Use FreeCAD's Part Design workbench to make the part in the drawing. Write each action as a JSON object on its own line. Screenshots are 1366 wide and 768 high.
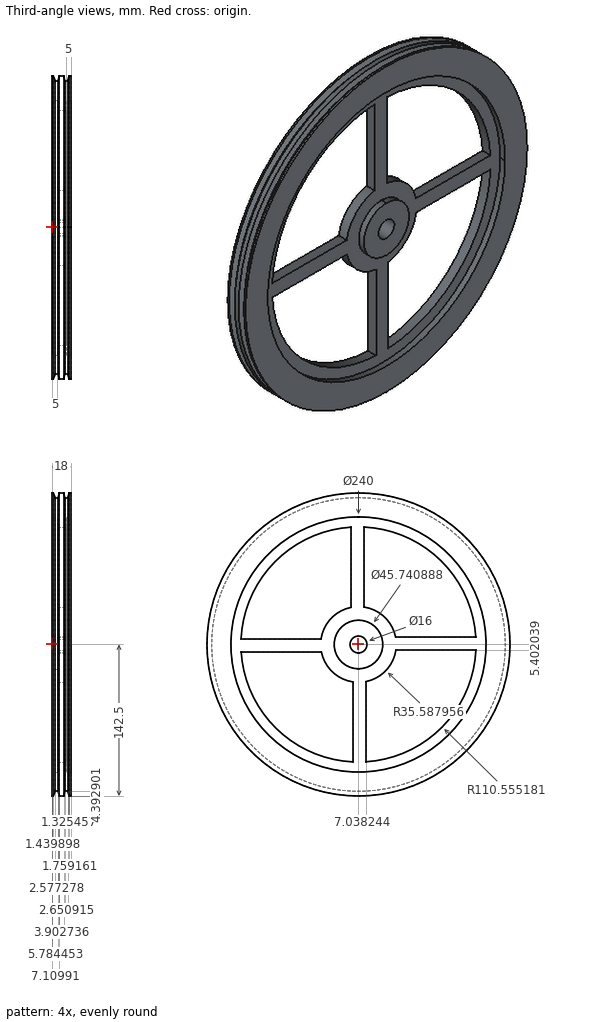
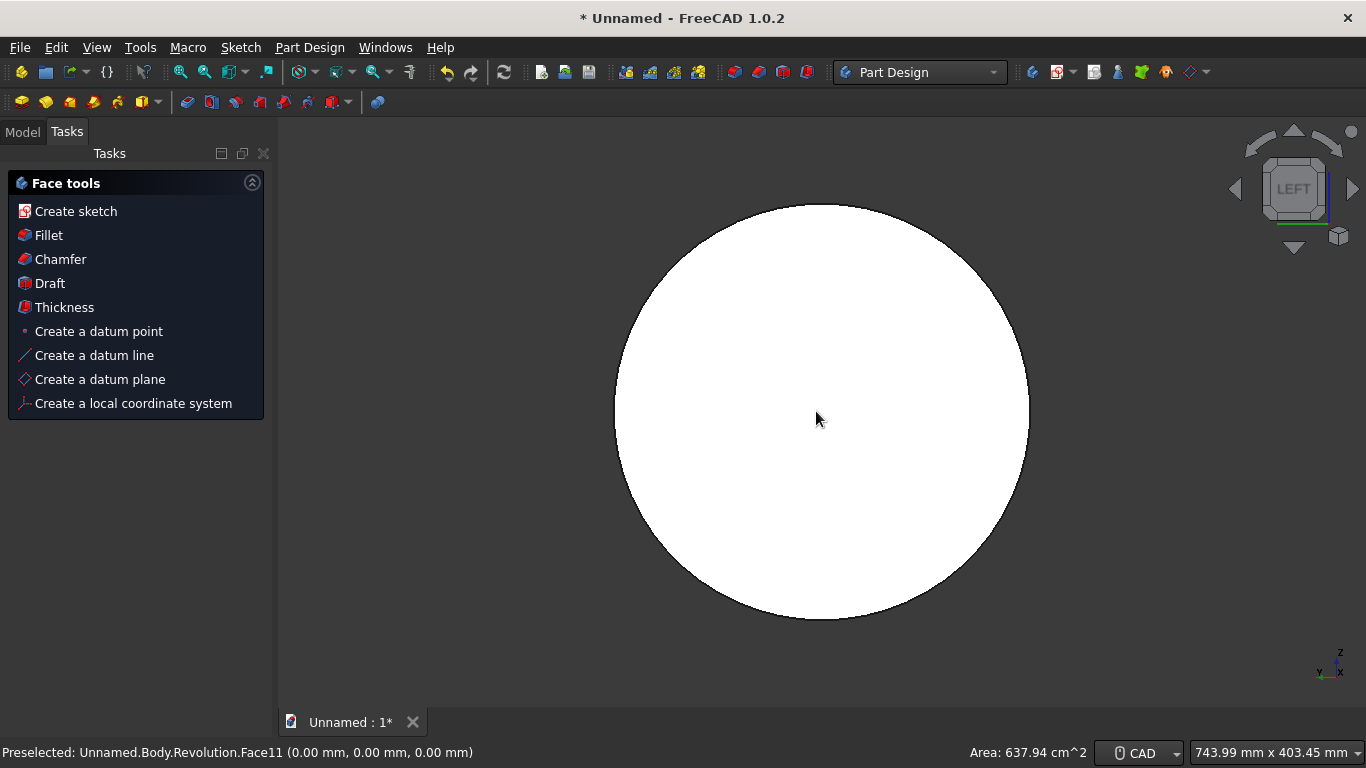
{"action": "left_click", "coordinate": [1058, 72]}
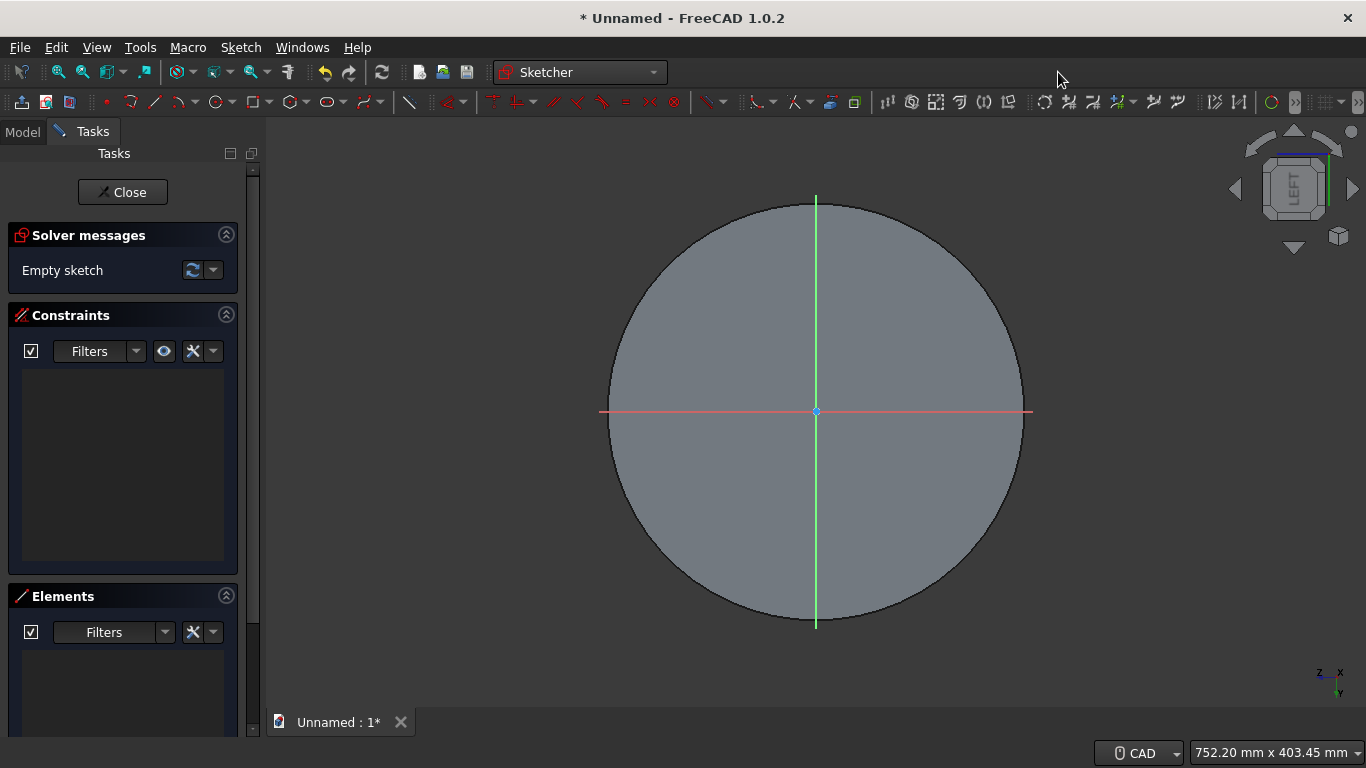
{"action": "key", "text": "g c"}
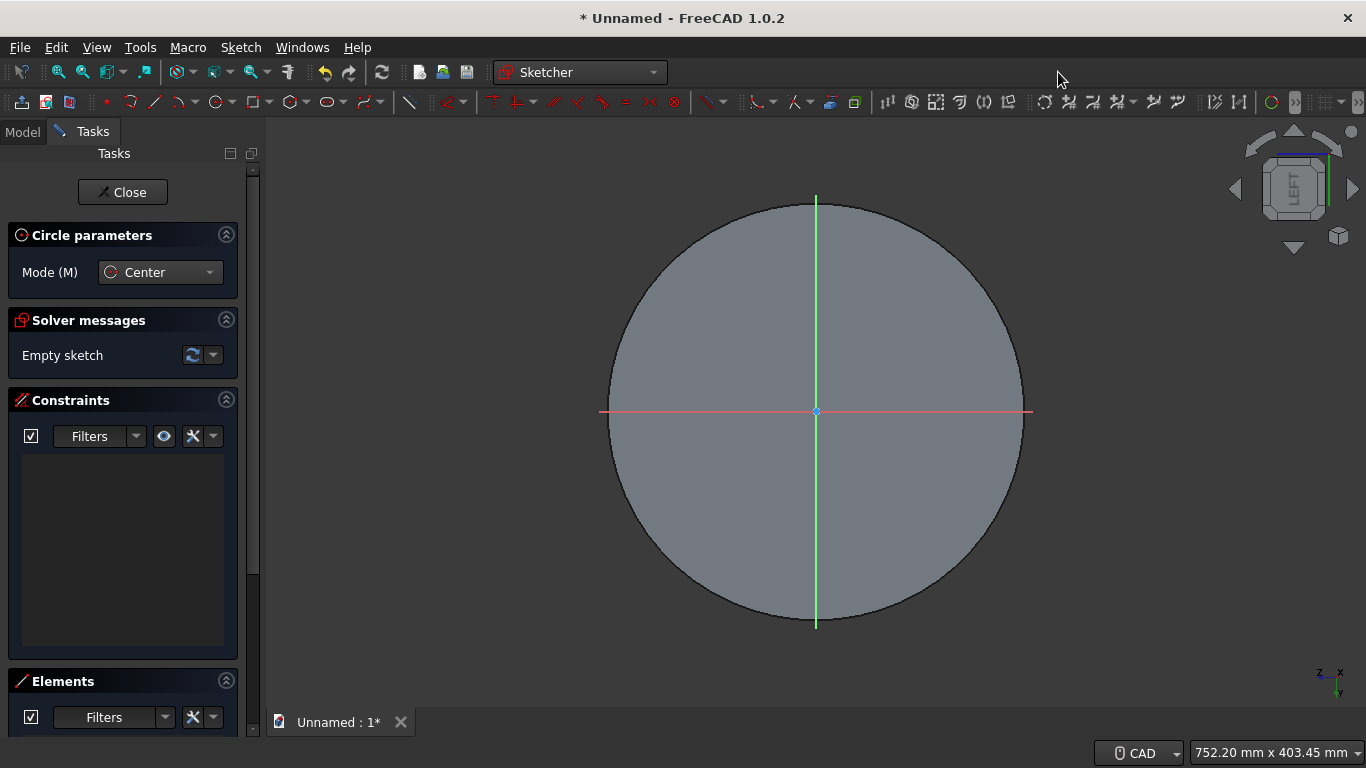
{"action": "left_click", "coordinate": [816, 412]}
{"action": "mouse_move", "coordinate": [940, 288]}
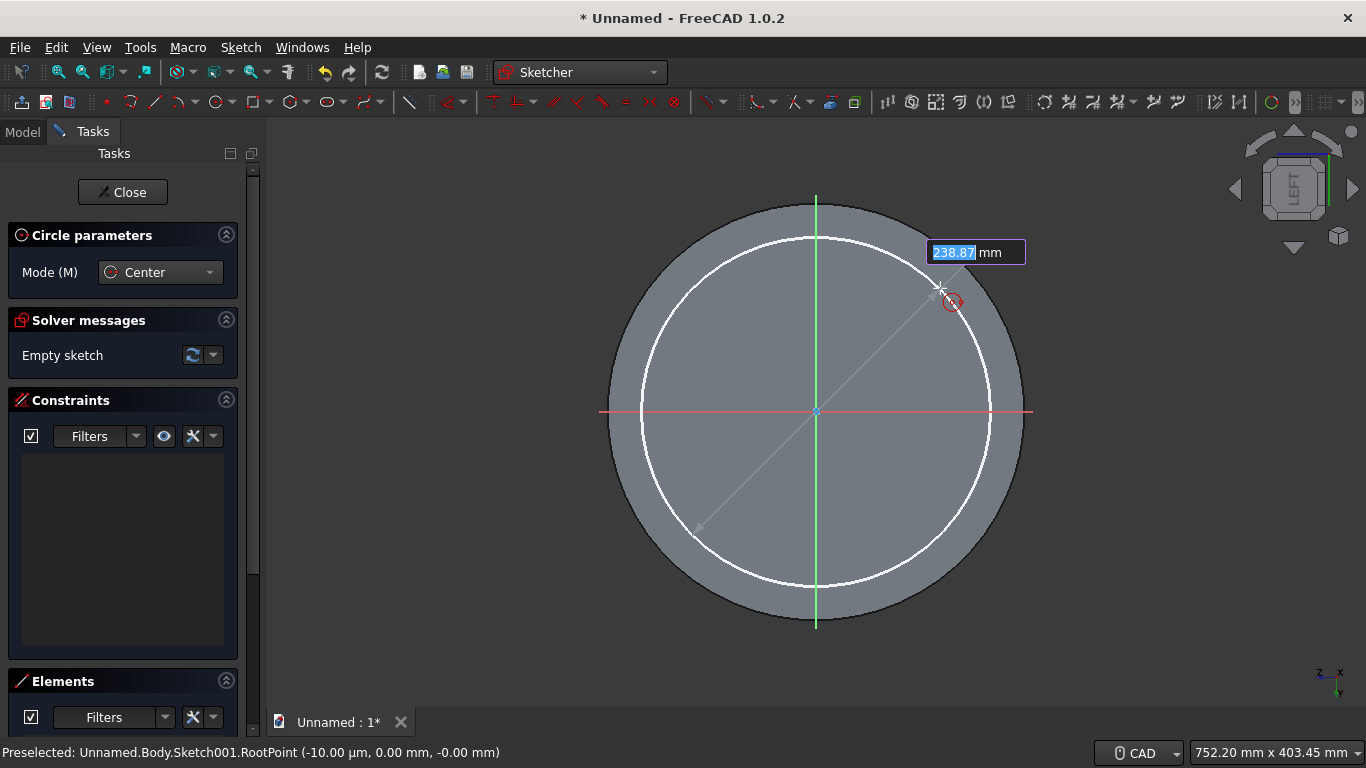
{"action": "type", "text": "240"}
{"action": "key", "text": "Return"}
{"action": "key", "text": "Escape"}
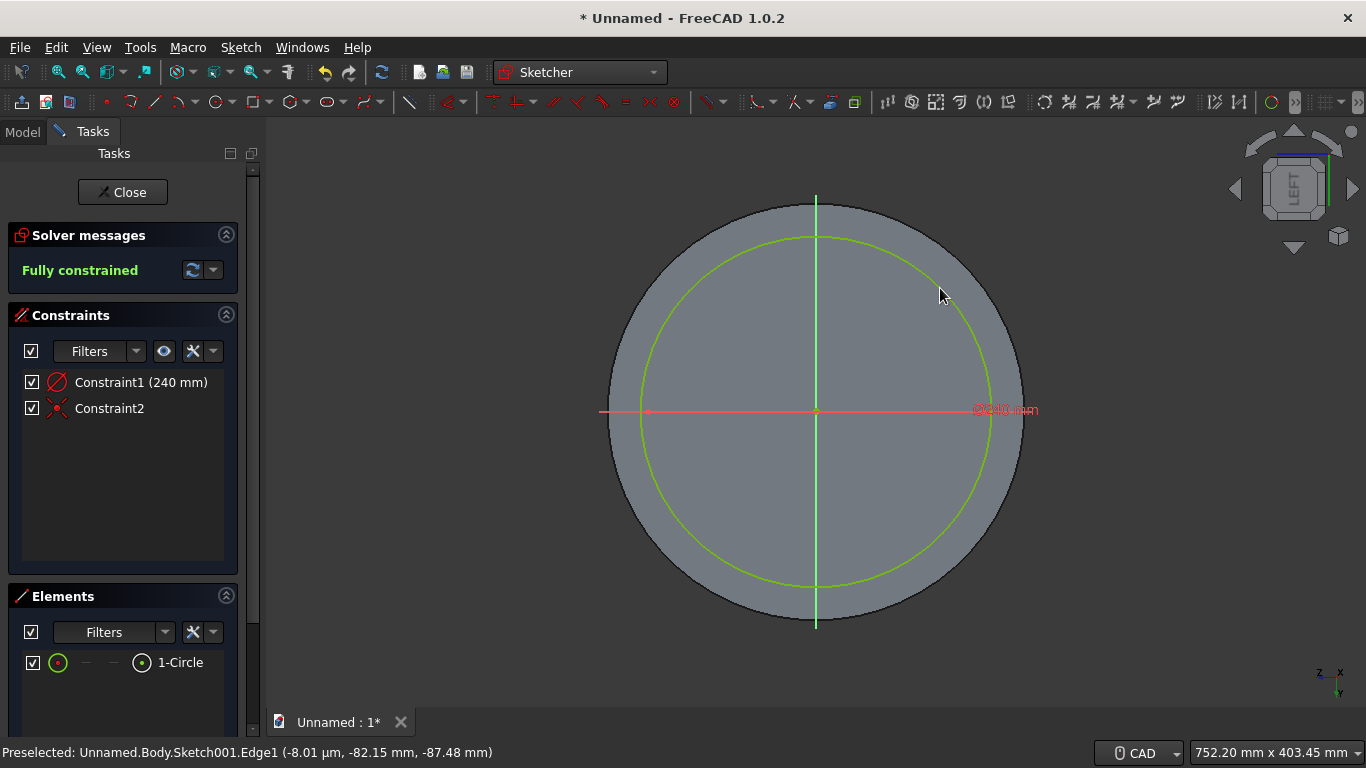
{"action": "left_click", "coordinate": [123, 192]}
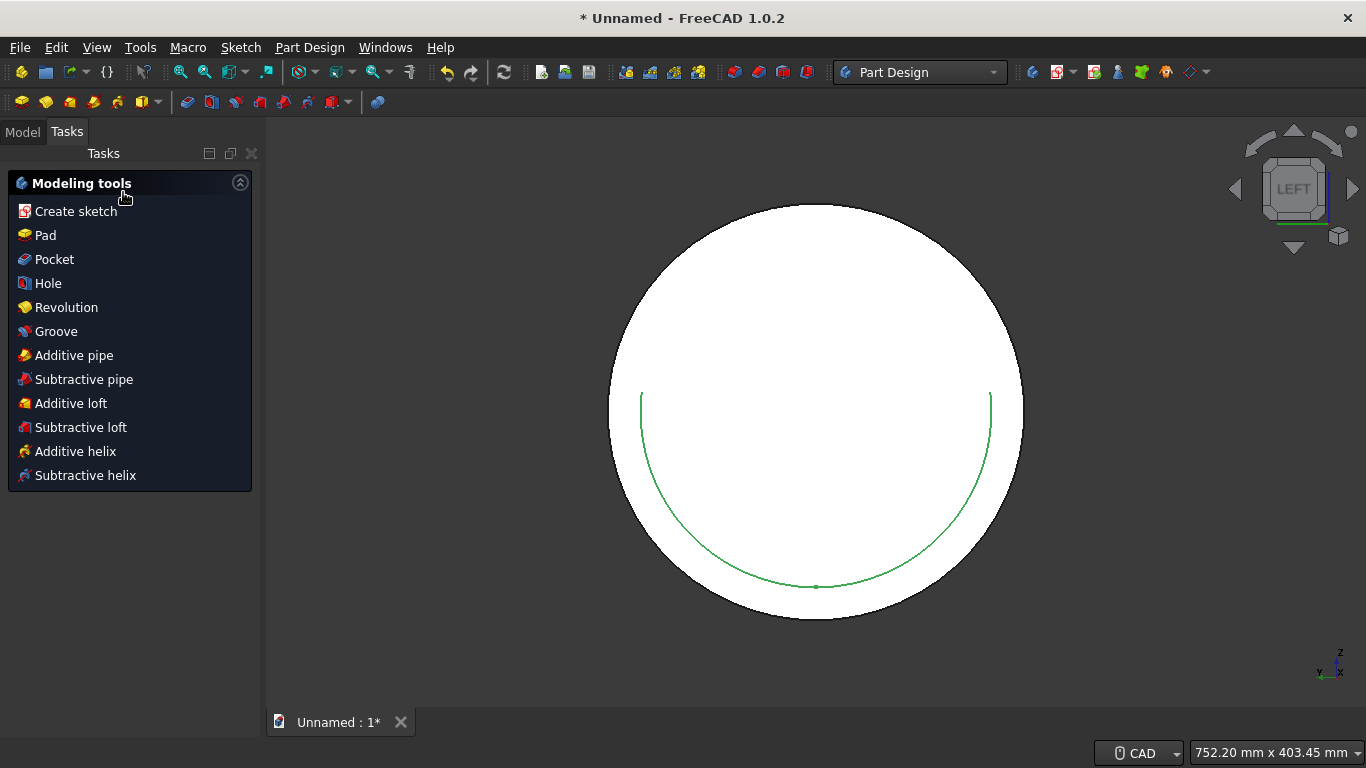
{"action": "left_click", "coordinate": [188, 102]}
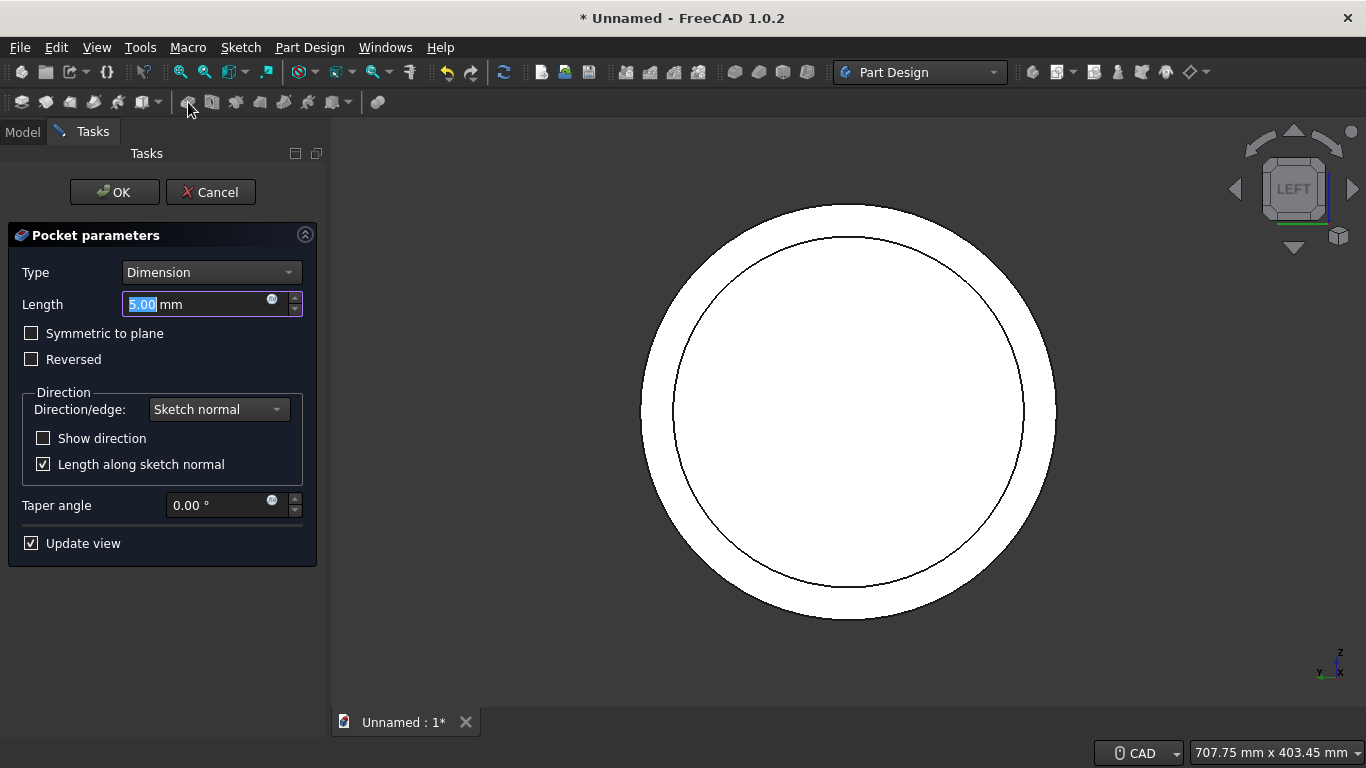
{"action": "type", "text": "5"}
{"action": "key", "text": "Tab"}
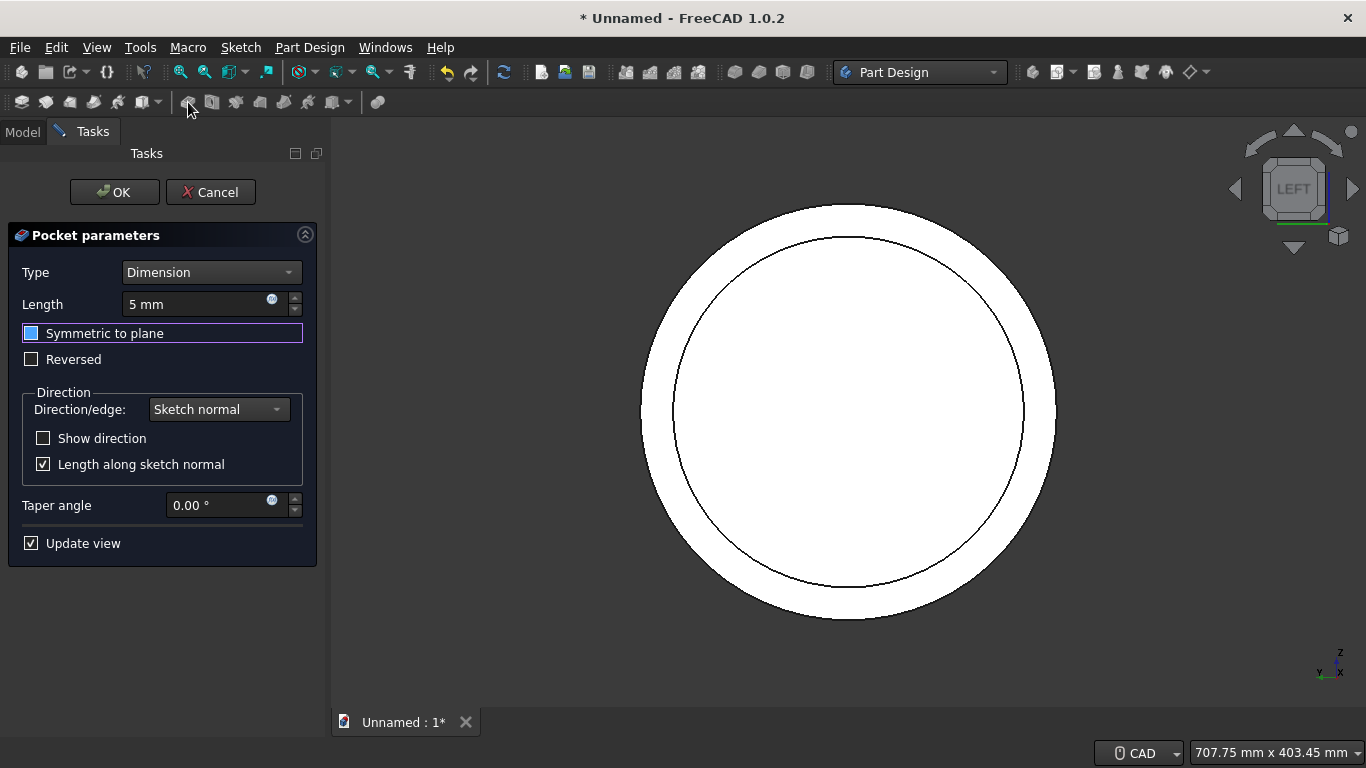
{"action": "left_click", "coordinate": [115, 192]}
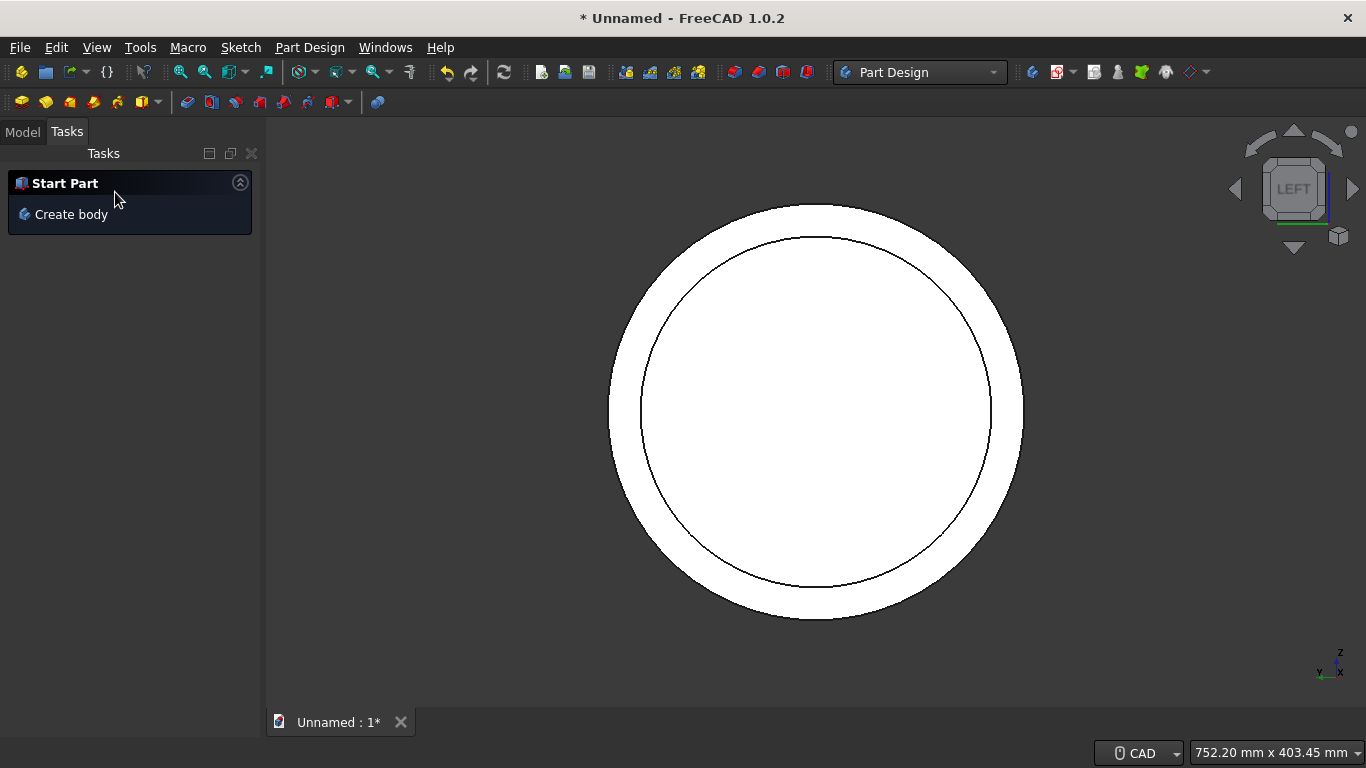
{"action": "left_click", "coordinate": [23, 131]}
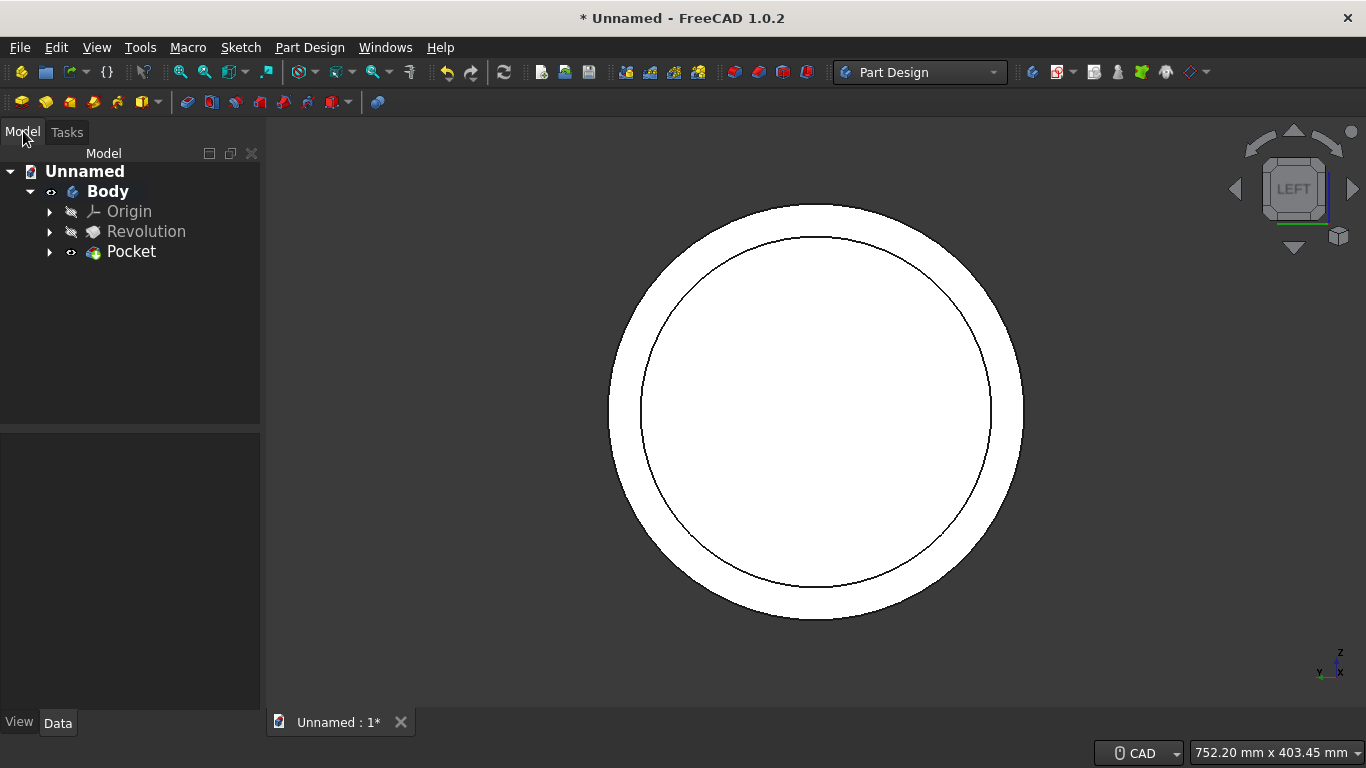
{"action": "left_click", "coordinate": [50, 212]}